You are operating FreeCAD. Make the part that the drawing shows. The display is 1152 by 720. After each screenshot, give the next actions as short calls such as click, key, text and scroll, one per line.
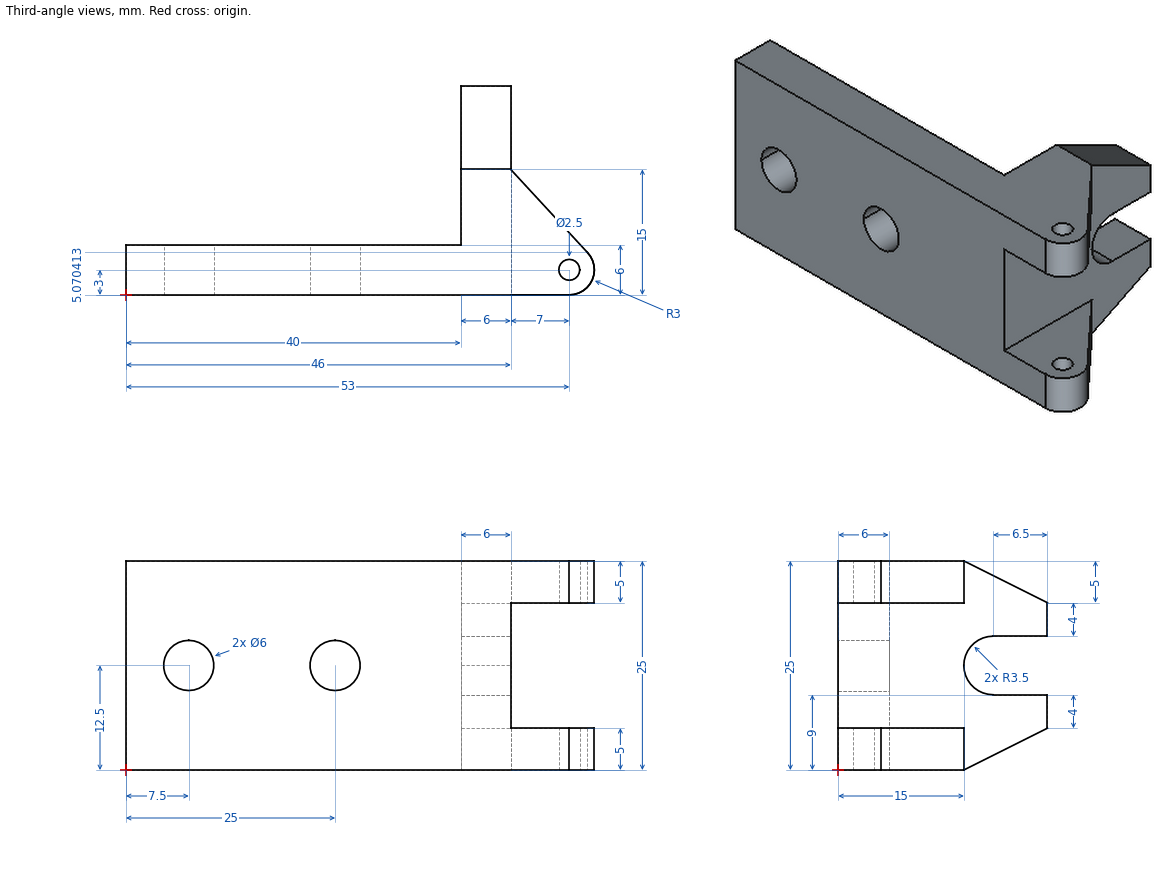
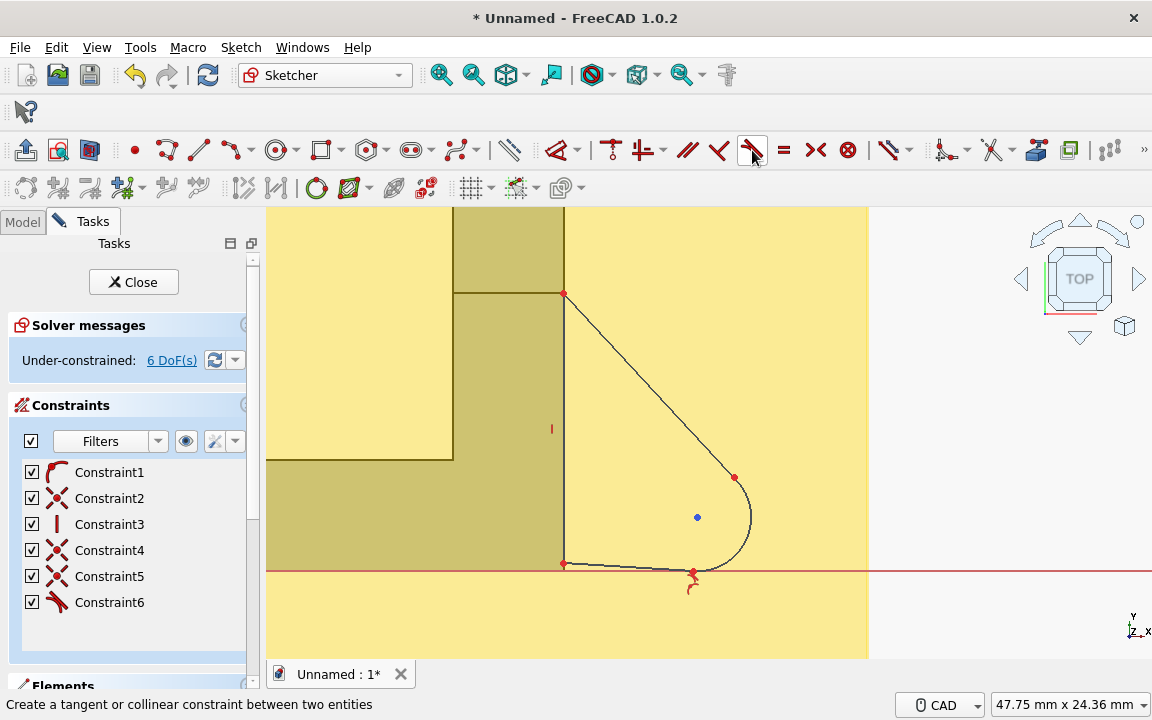
click(655, 569)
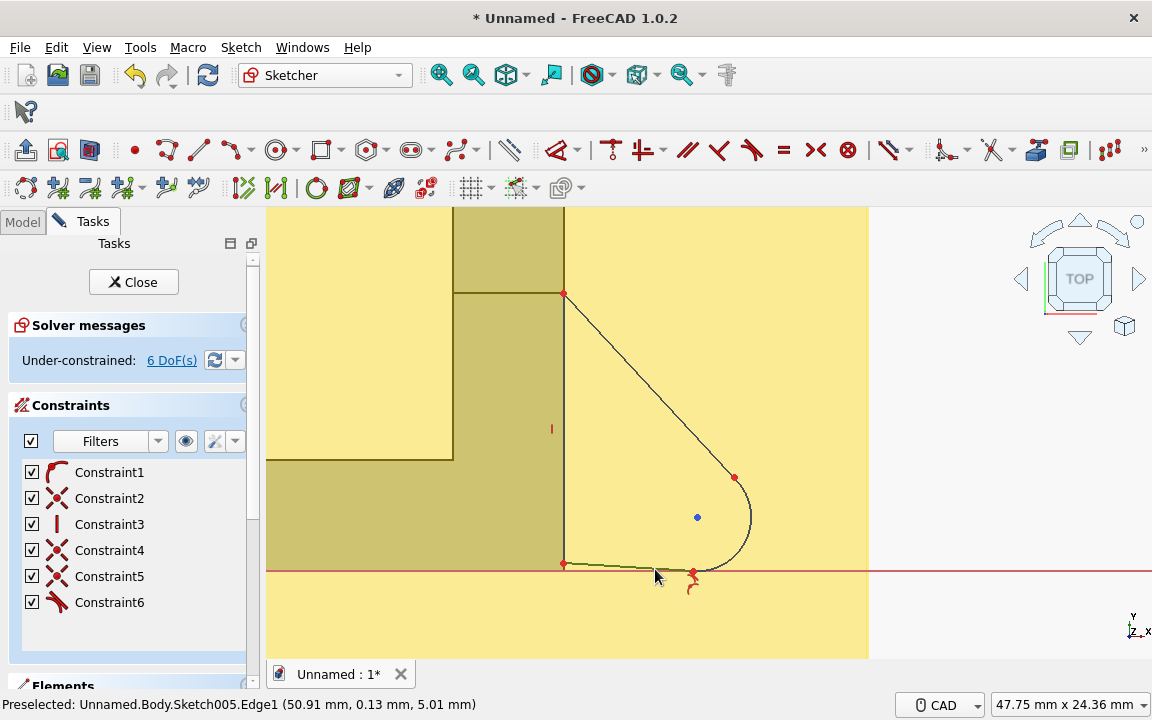
key(h)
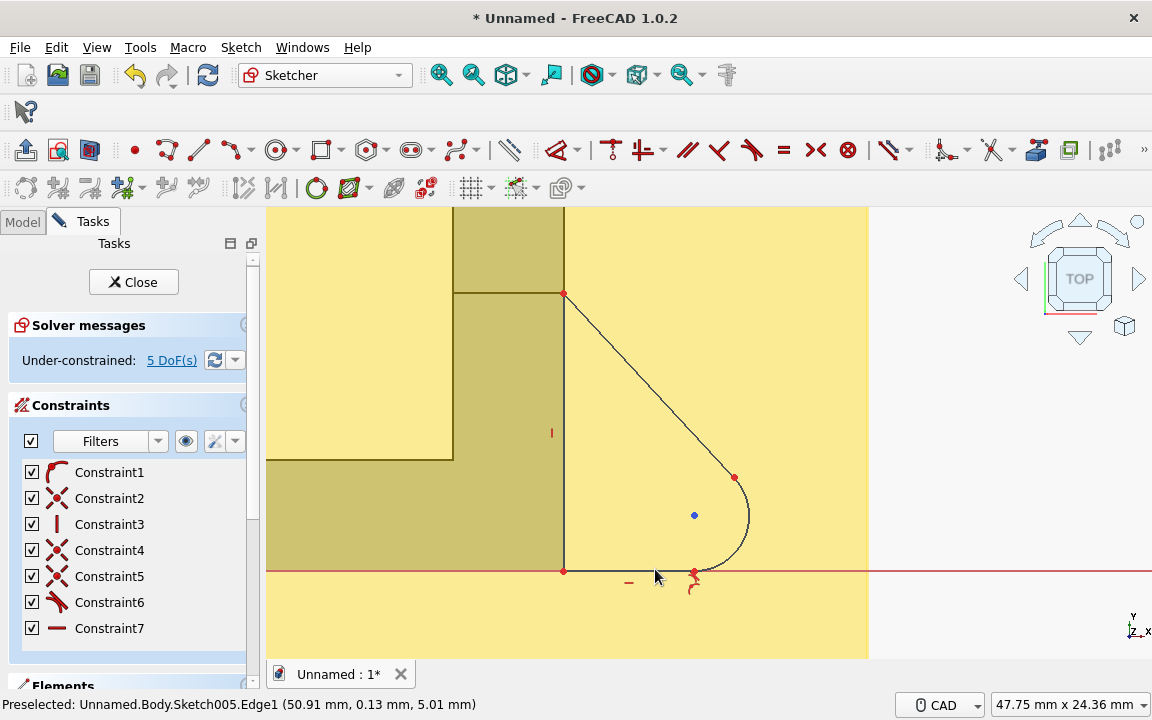
key(d)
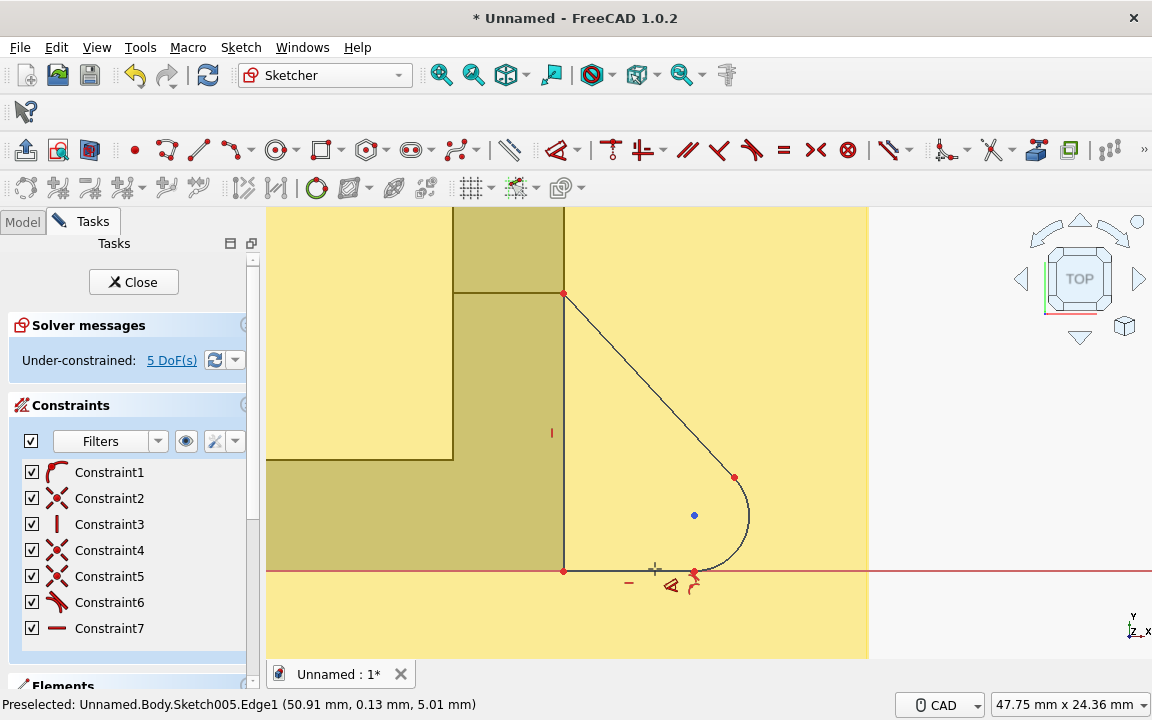
click(729, 558)
click(711, 601)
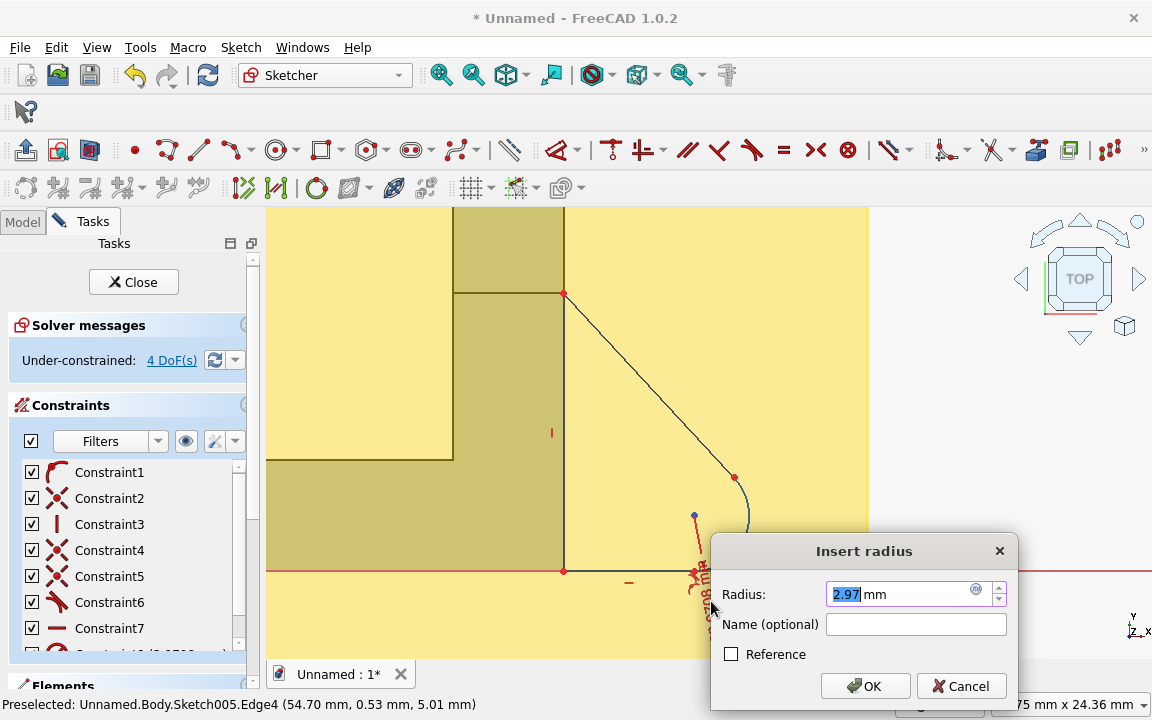
text(3)
key(Return)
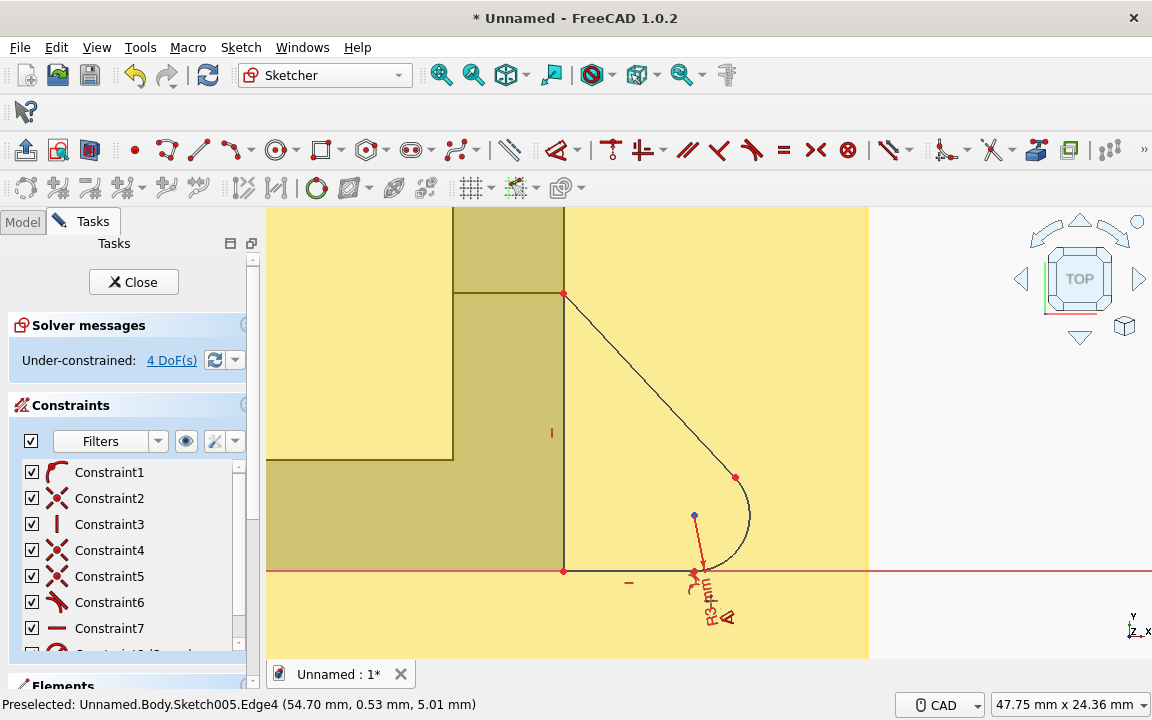
click(655, 571)
click(629, 605)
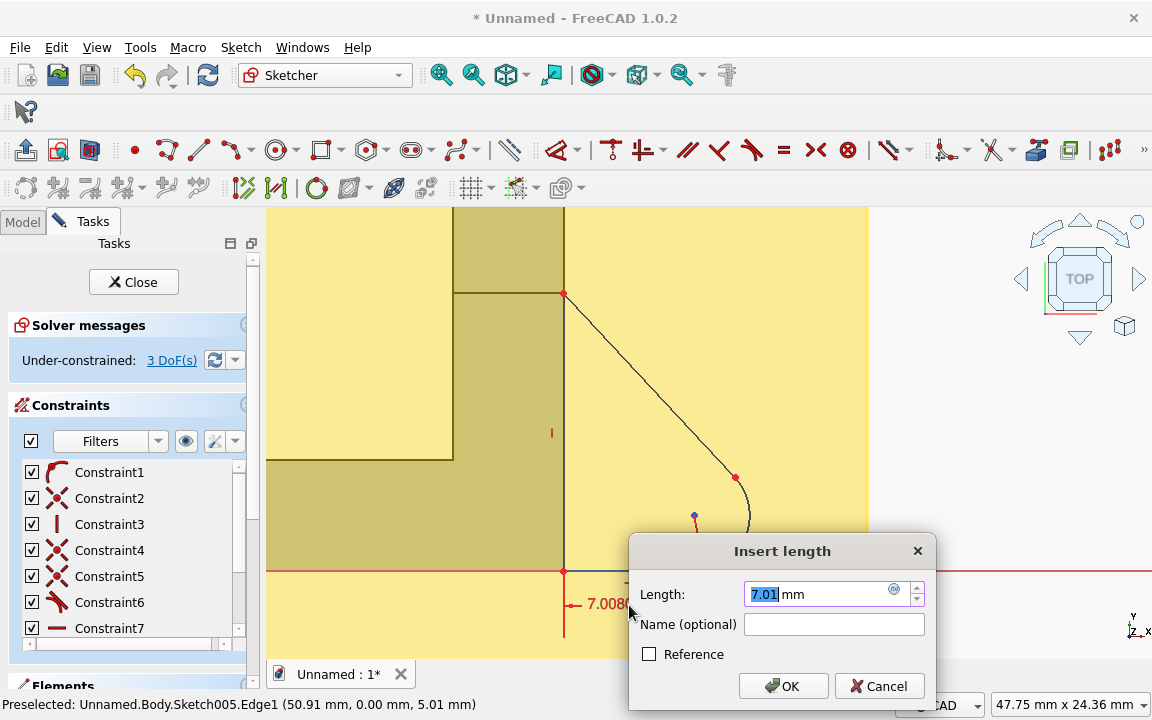
text(7)
key(Return)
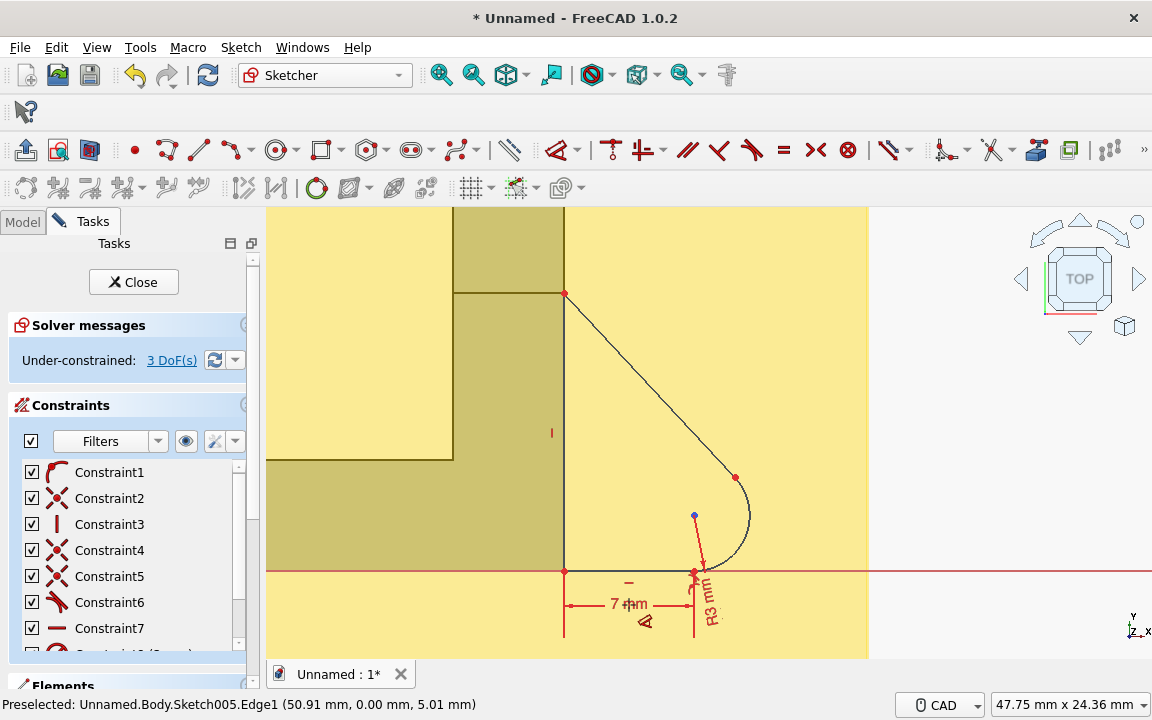
click(564, 488)
click(530, 433)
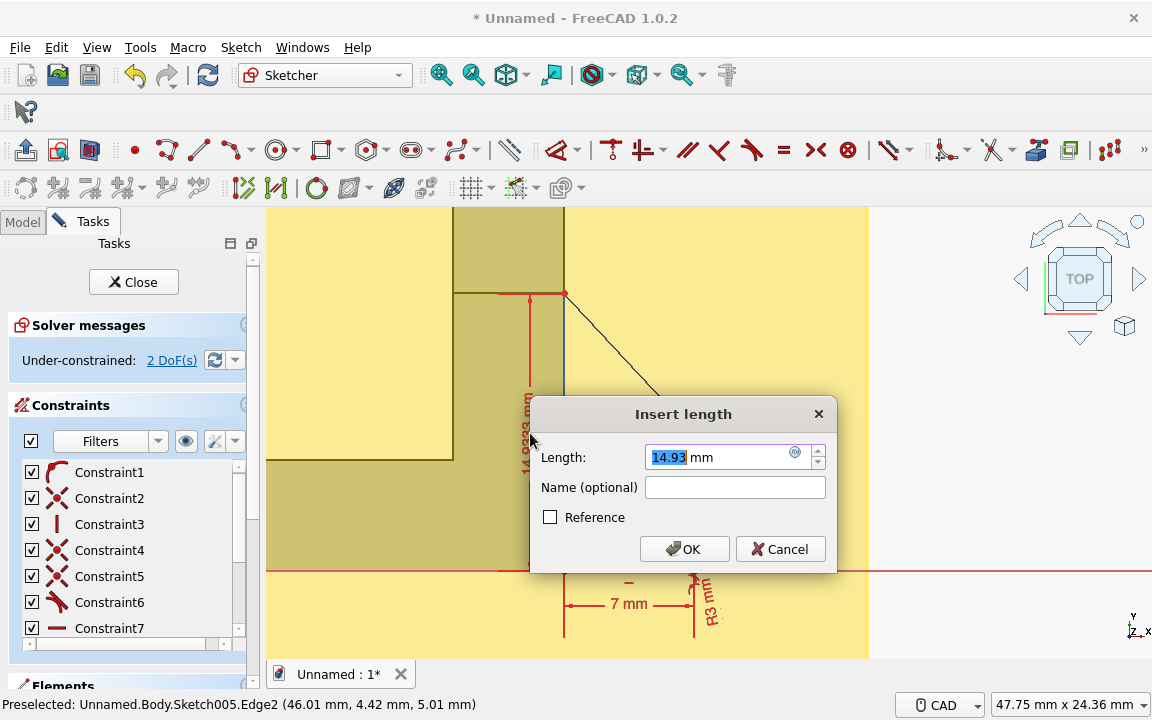
text(15)
key(Return)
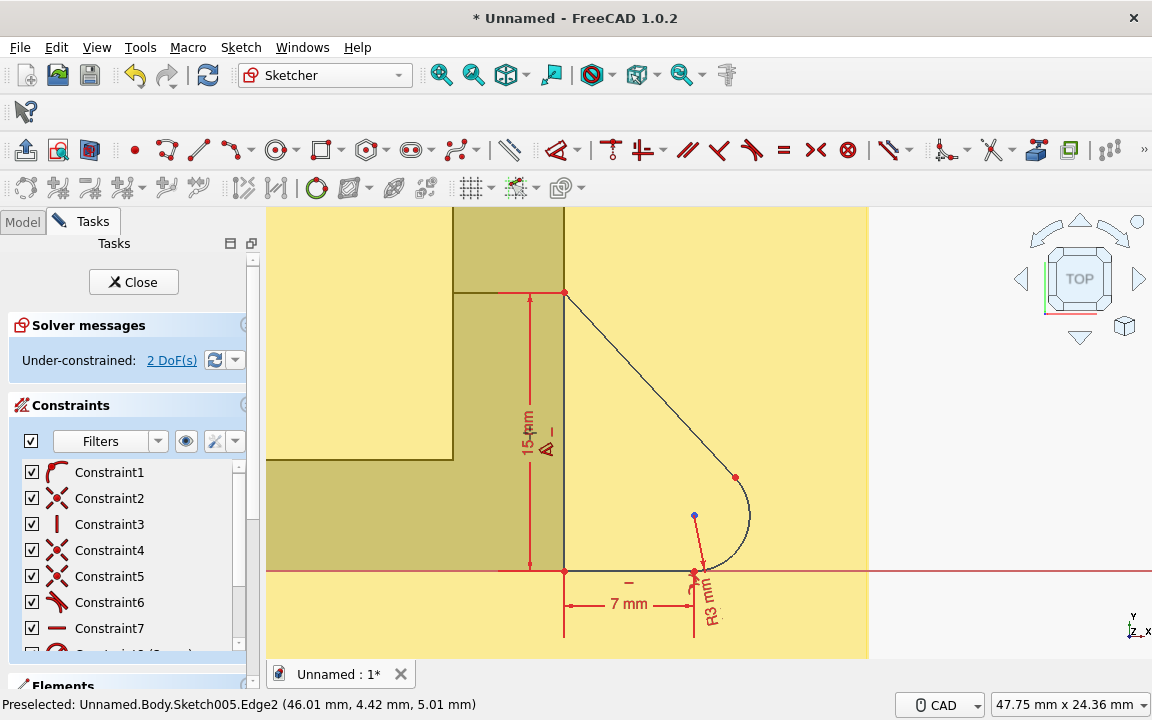
click(694, 571)
click(494, 605)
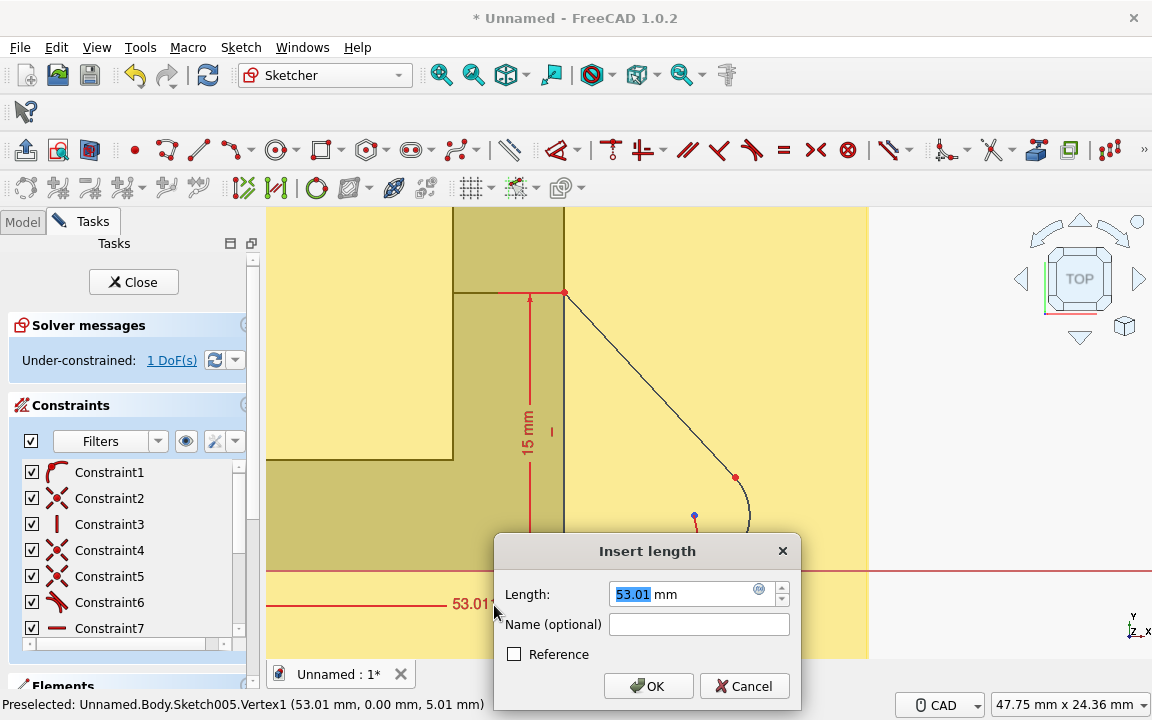
text(53)
key(Return)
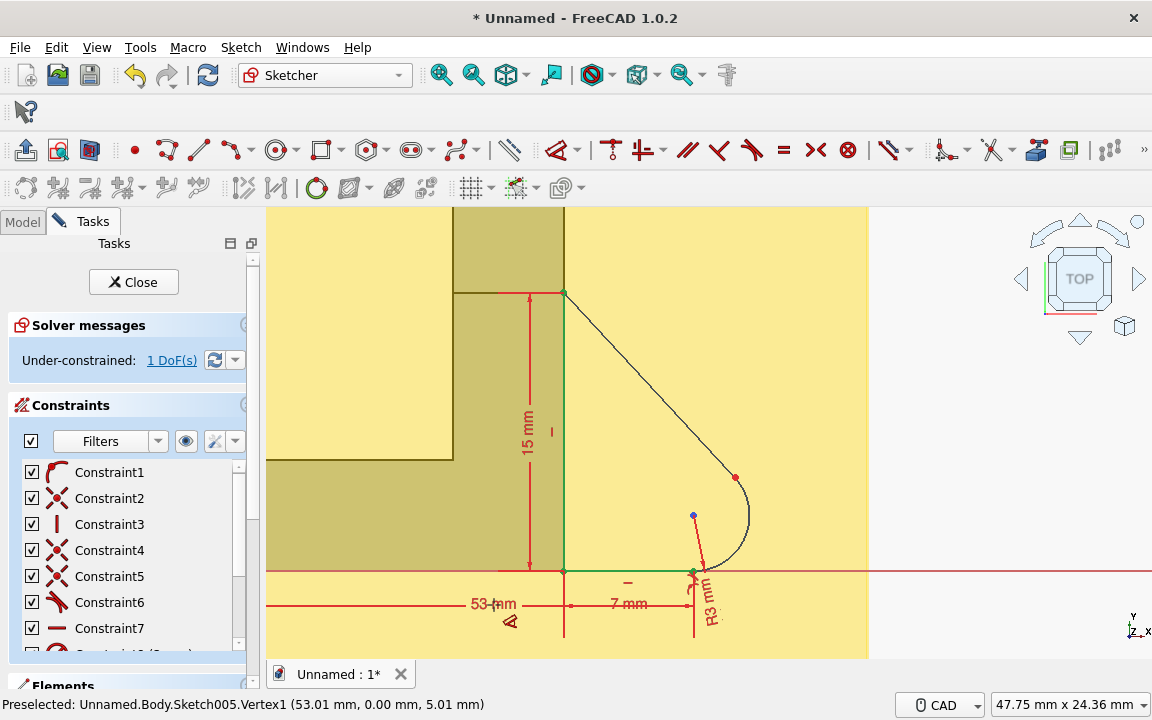
click(735, 478)
click(769, 525)